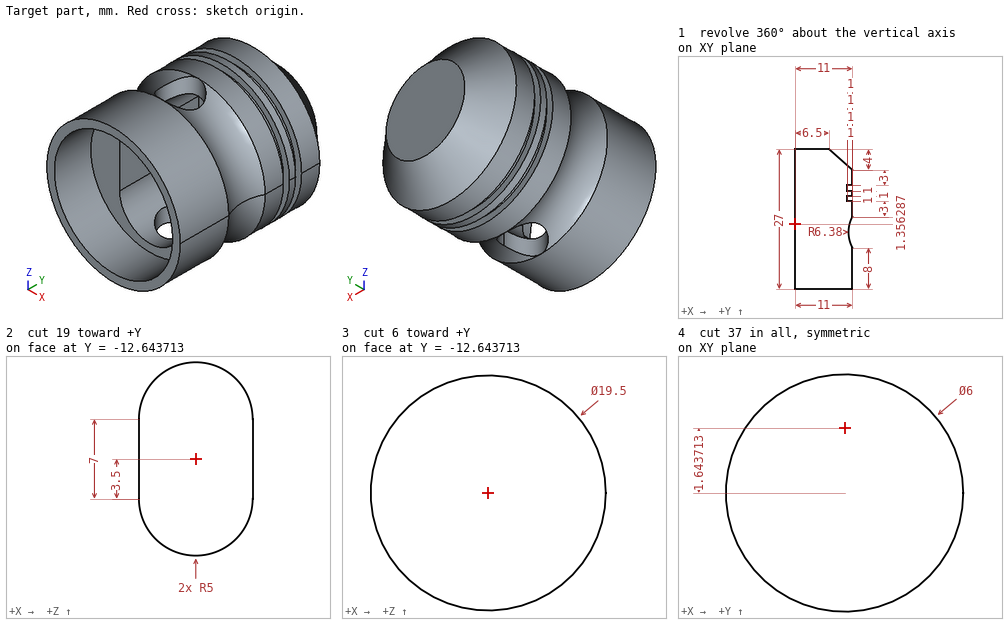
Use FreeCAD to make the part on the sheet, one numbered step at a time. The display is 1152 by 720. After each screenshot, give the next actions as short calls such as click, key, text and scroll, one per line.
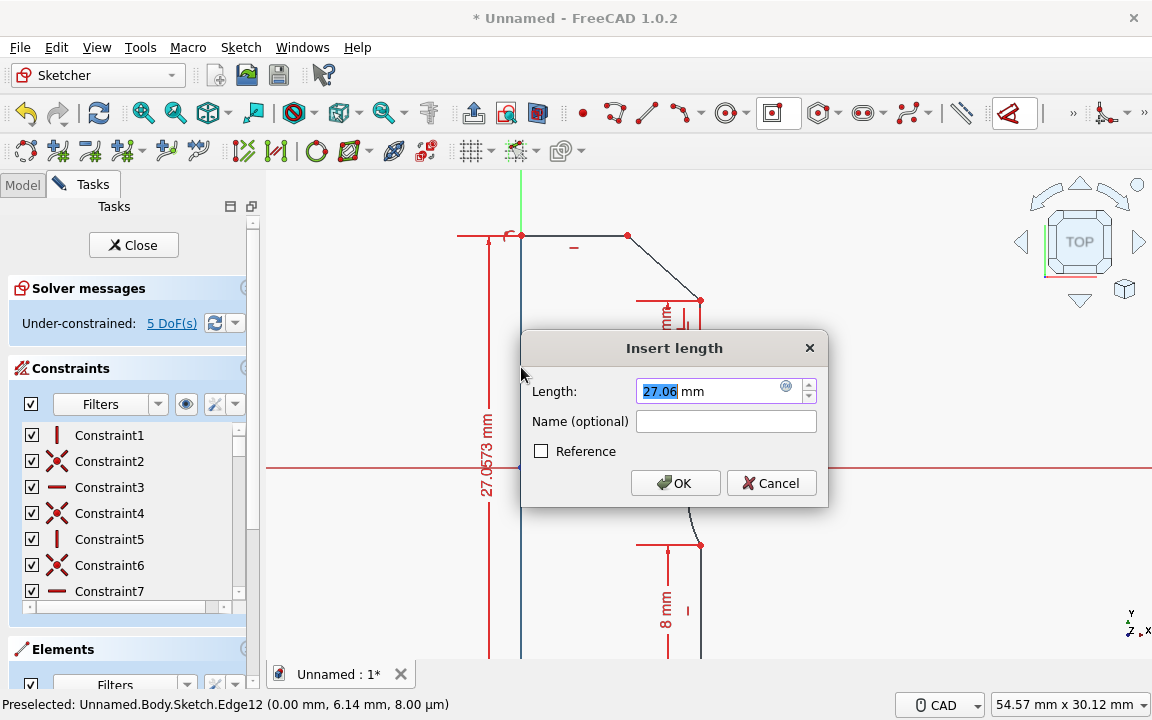
text(27)
key(Return)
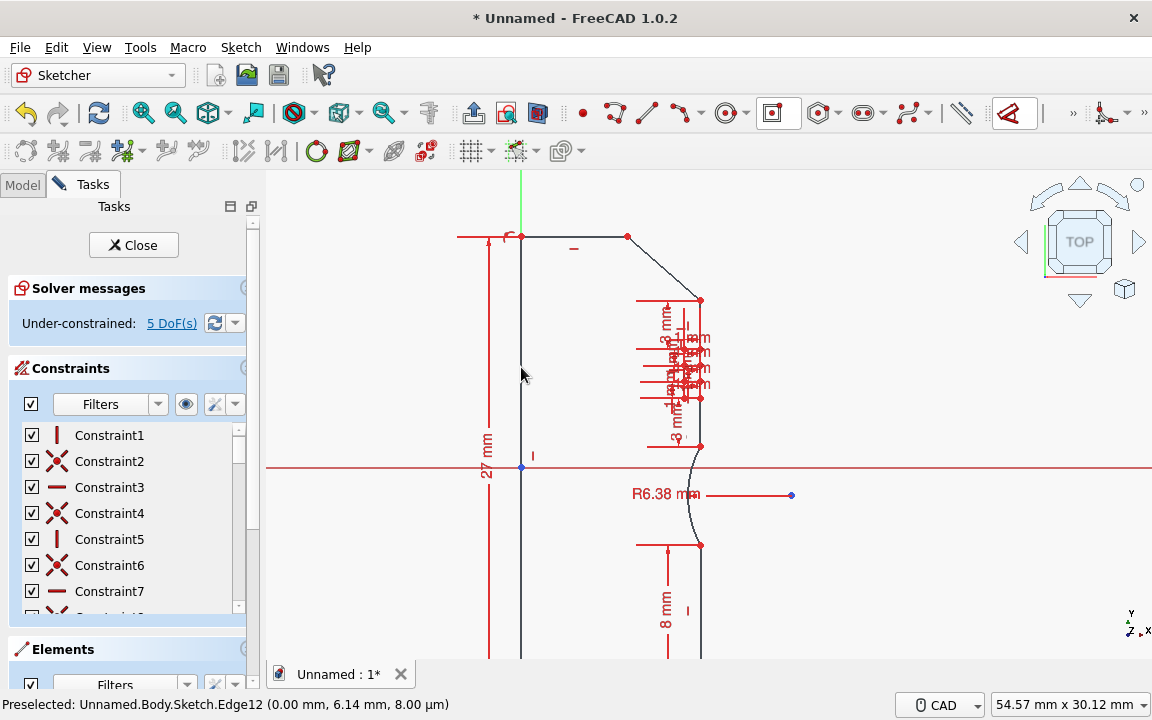
scroll(701, 334, down, 2)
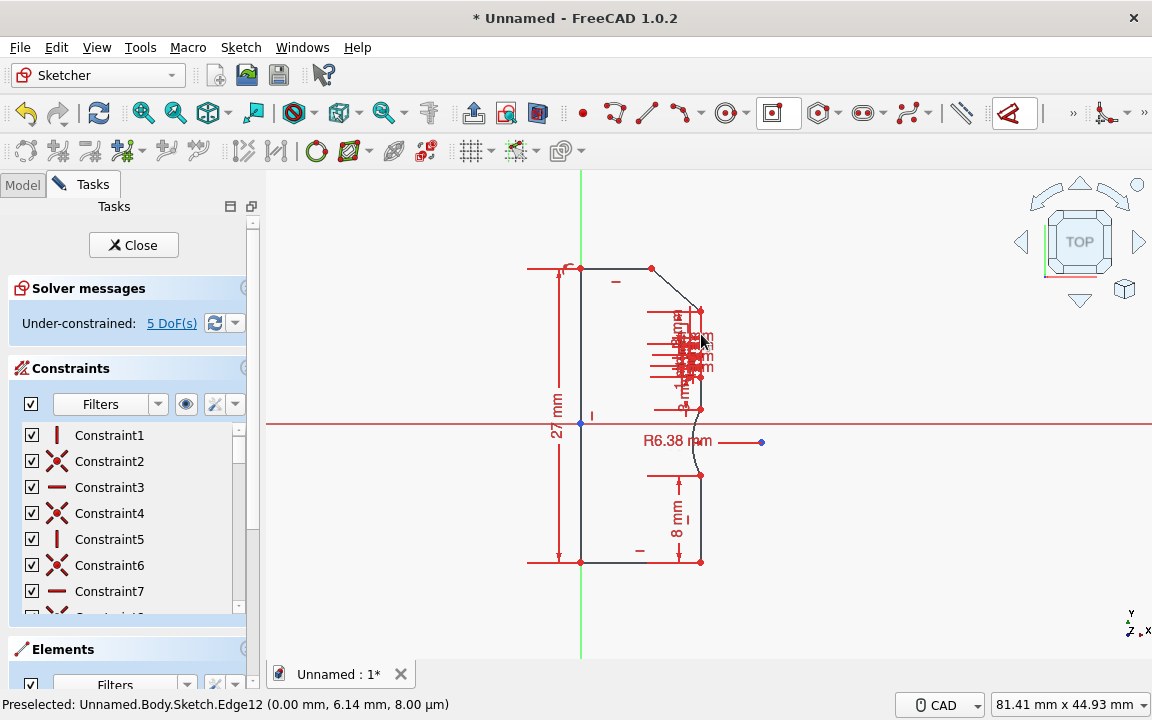
click(617, 563)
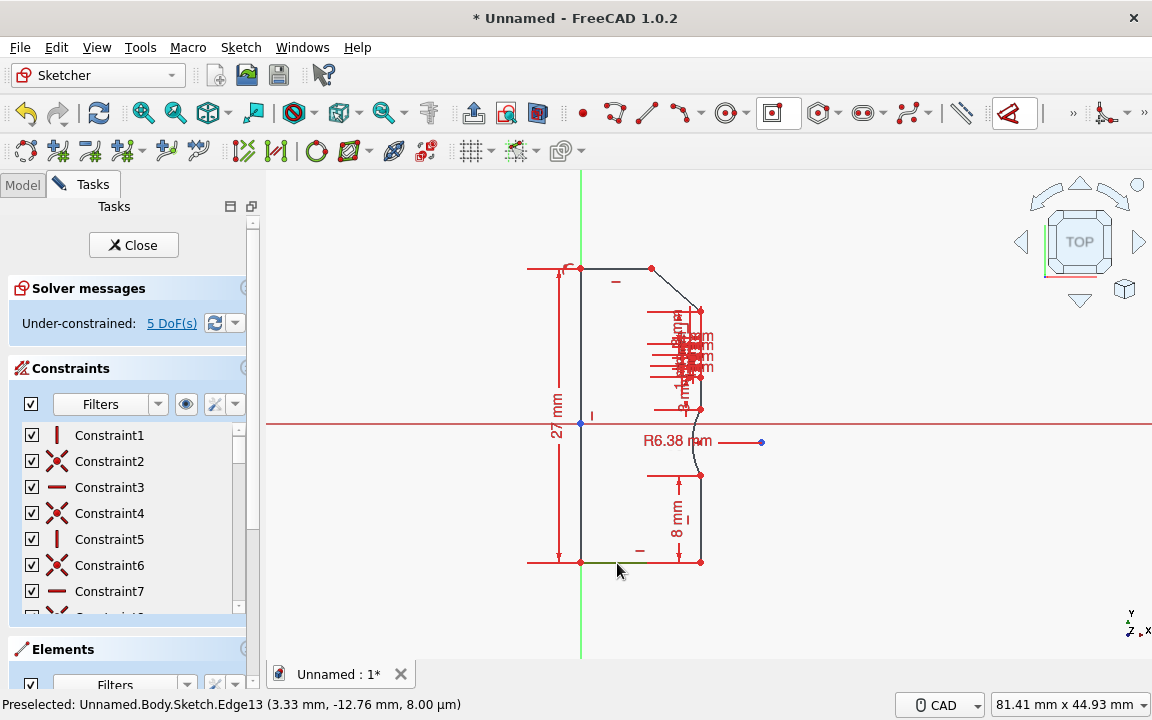
key(l)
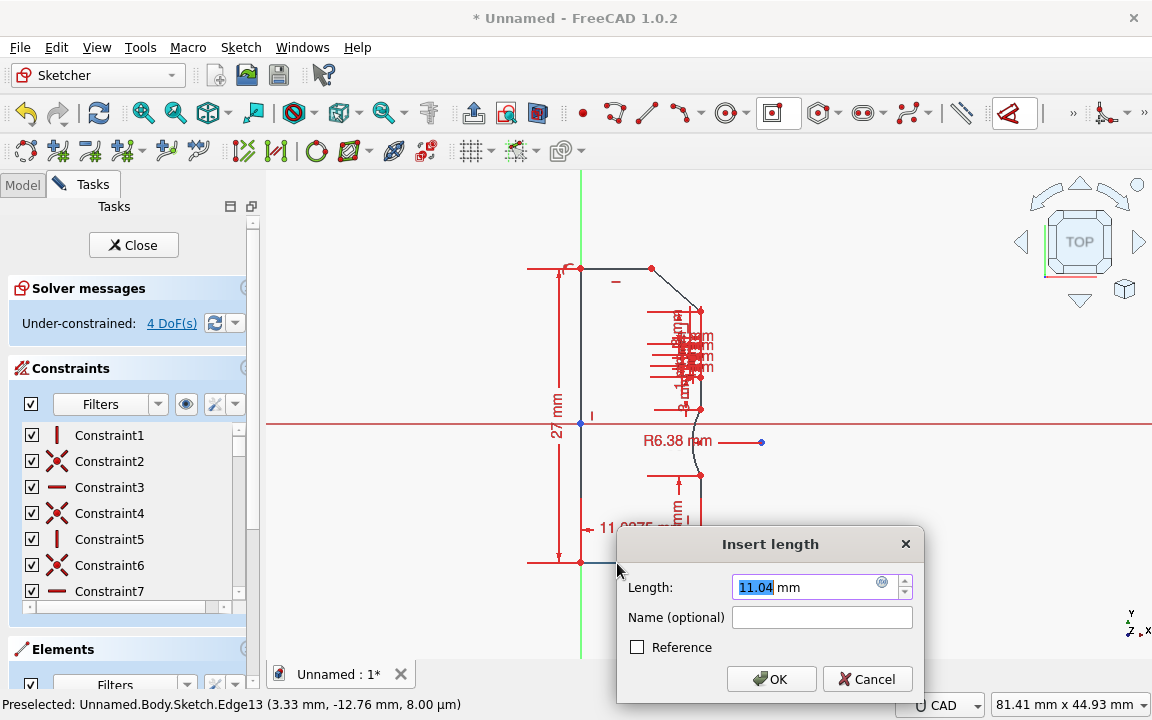
text(11)
key(Return)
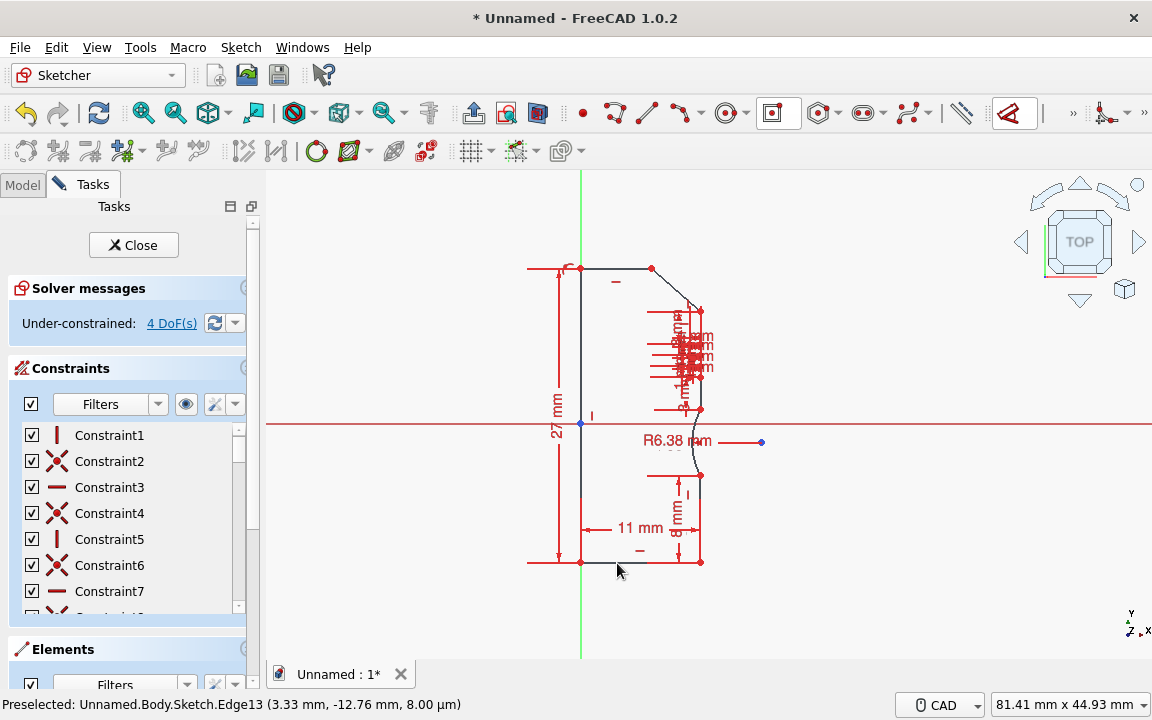
click(667, 282)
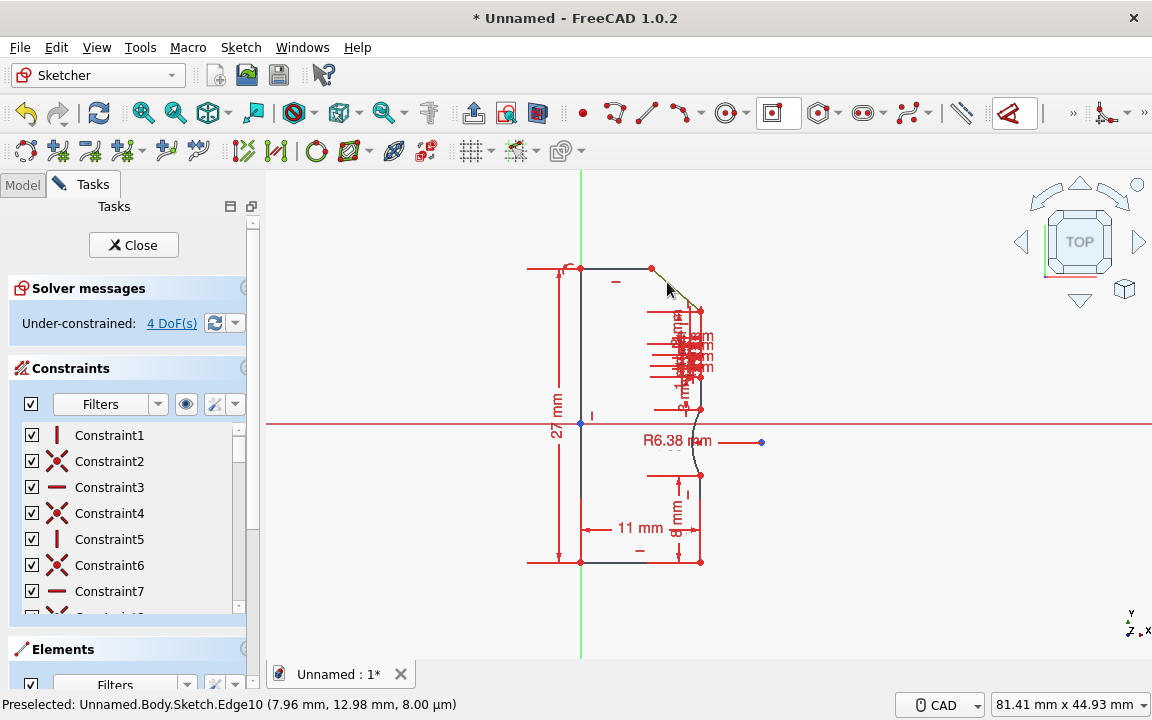
key(i)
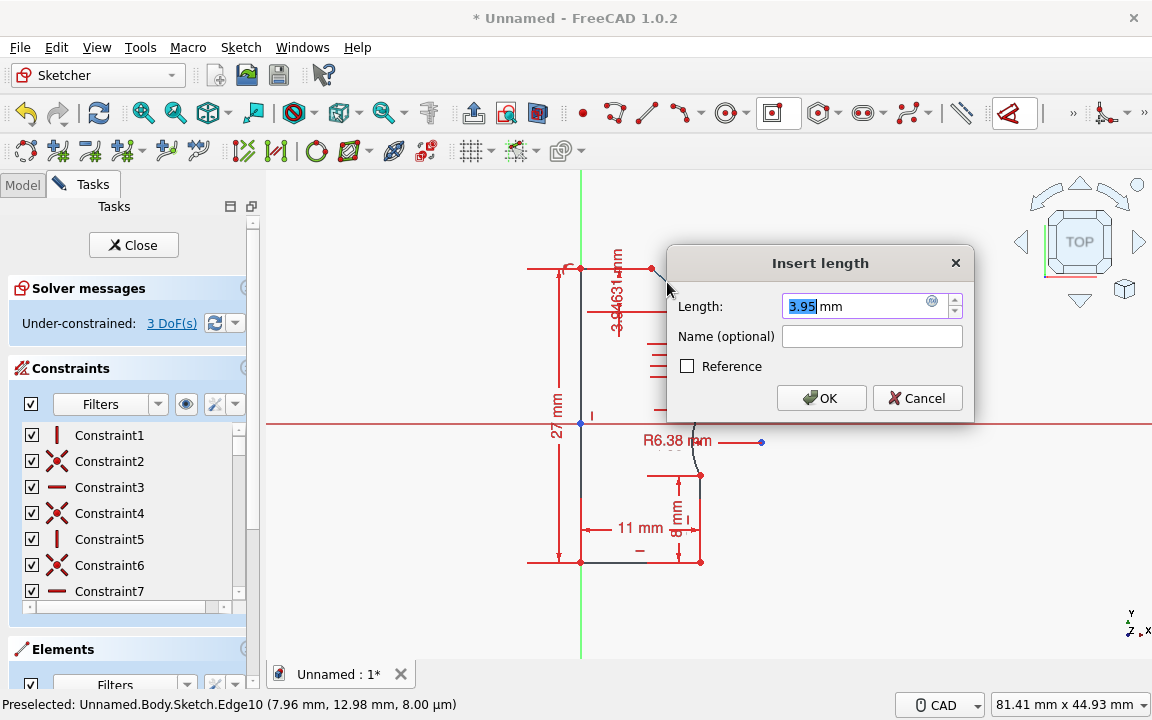
text(4)
key(Return)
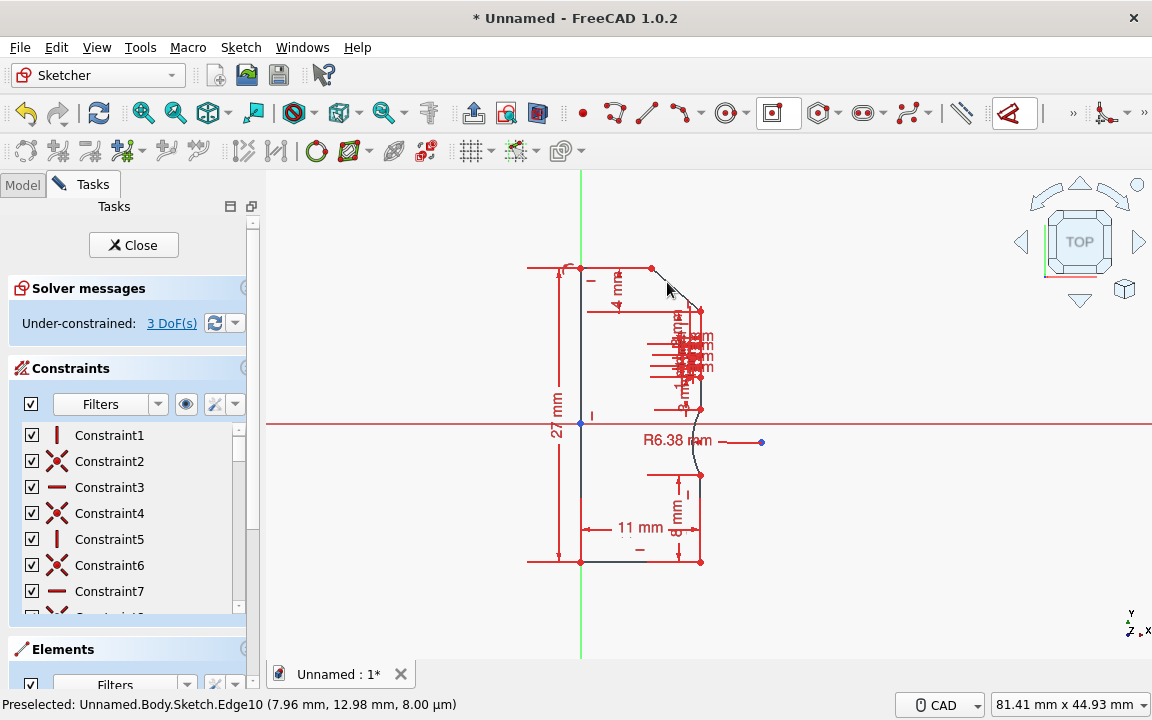
click(631, 268)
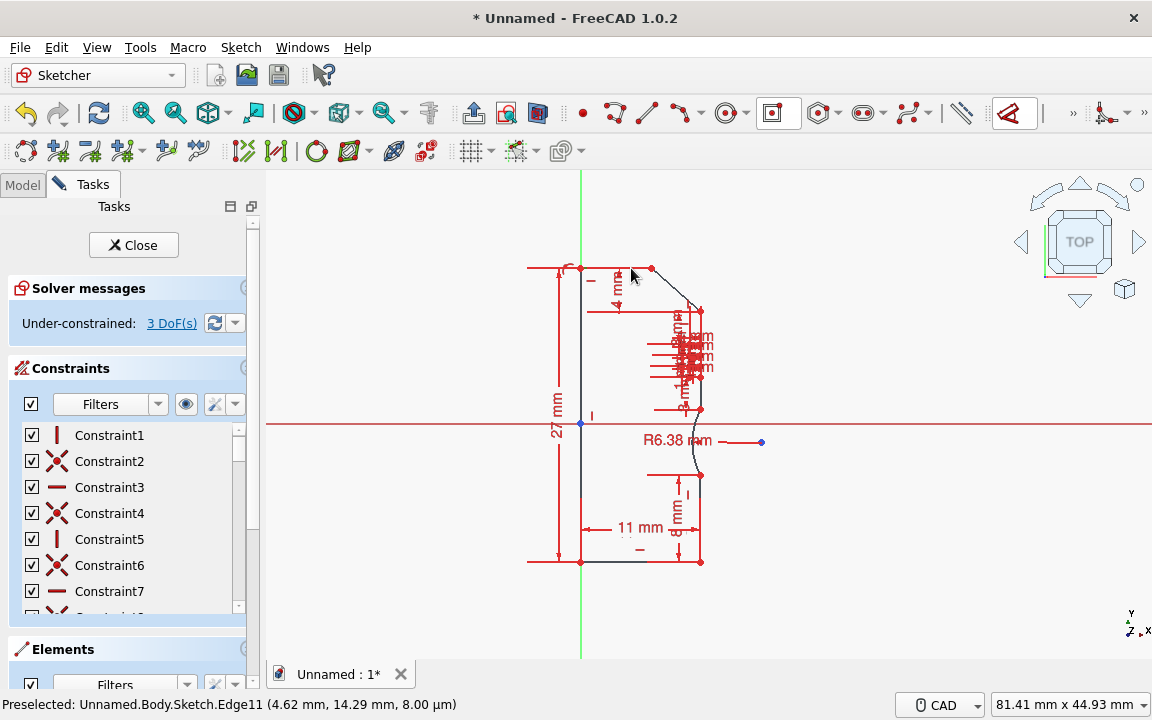
click(1032, 114)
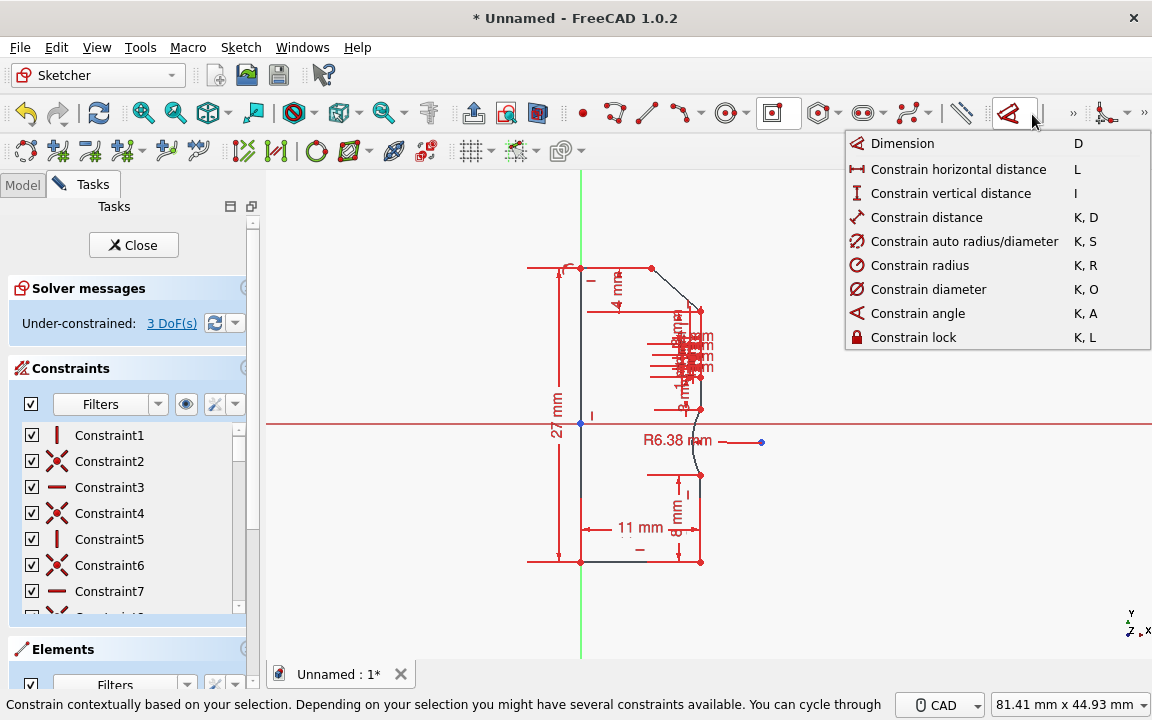
click(998, 169)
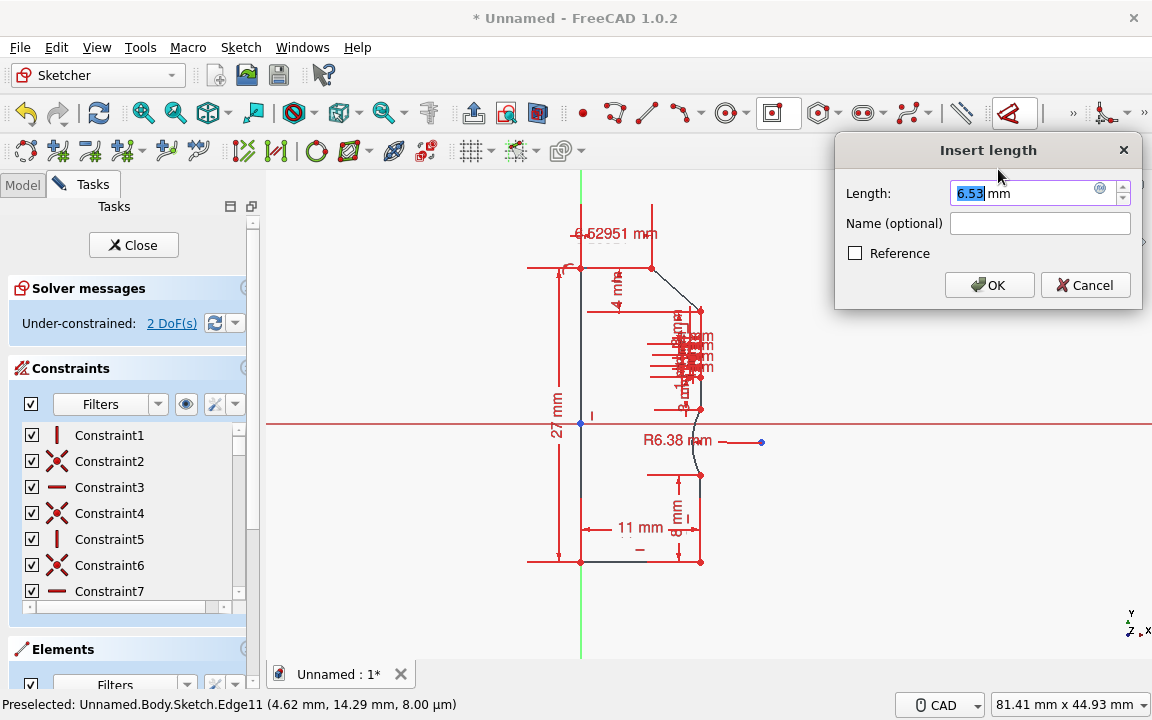
text(6.5)
key(Return)